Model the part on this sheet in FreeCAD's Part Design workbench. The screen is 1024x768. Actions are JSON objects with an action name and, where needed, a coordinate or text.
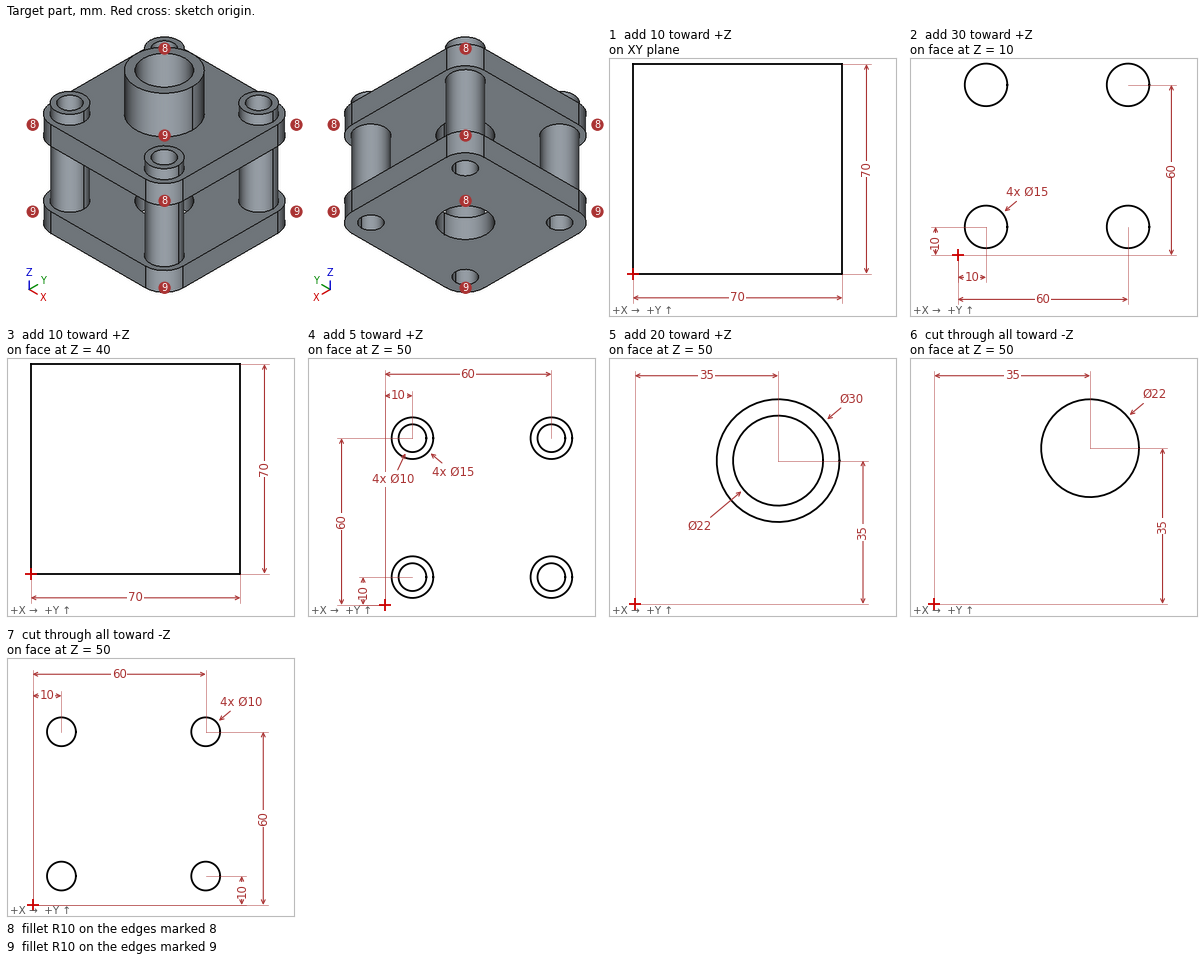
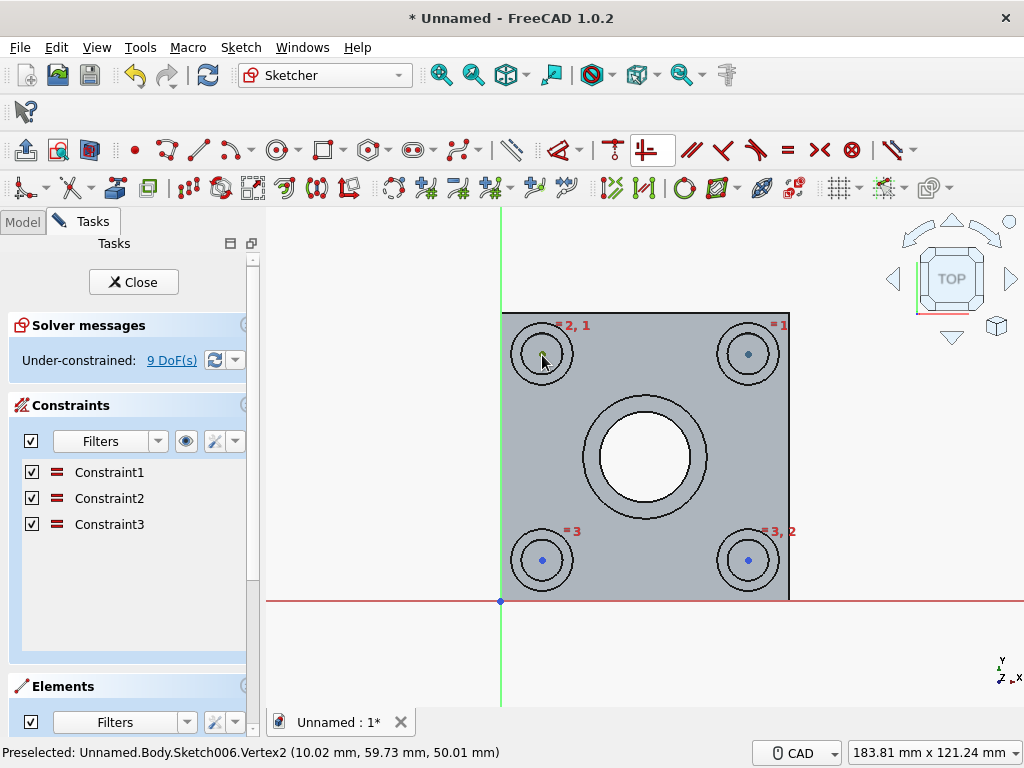
{"action": "key", "text": "h"}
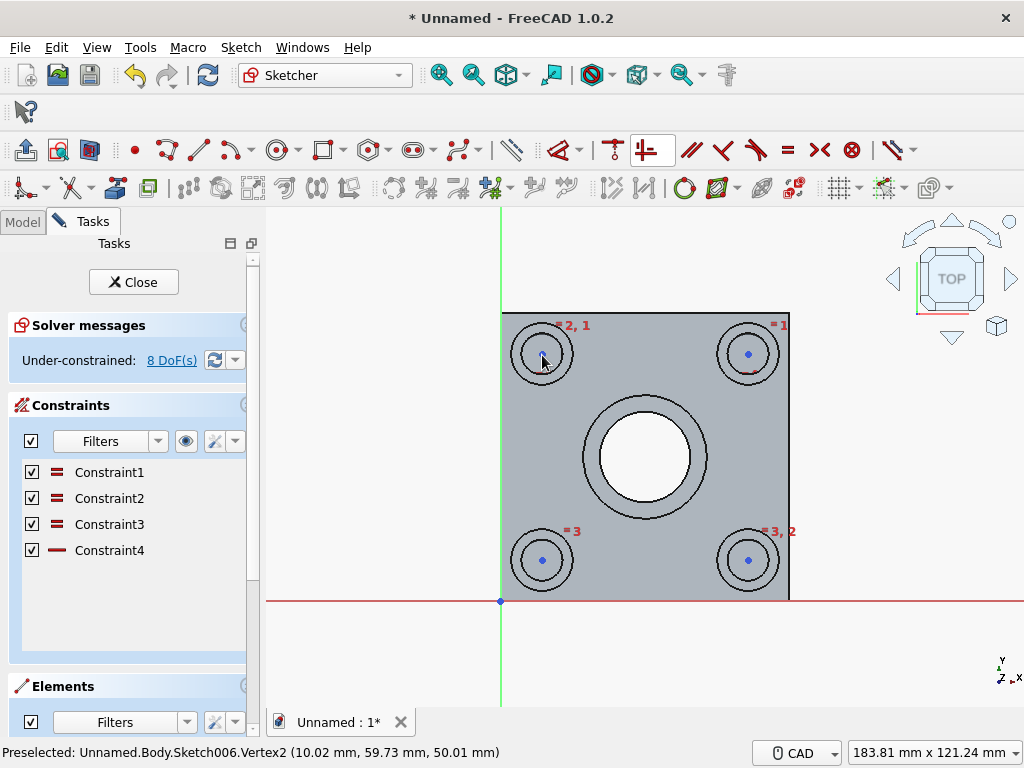
{"action": "left_click", "coordinate": [748, 355]}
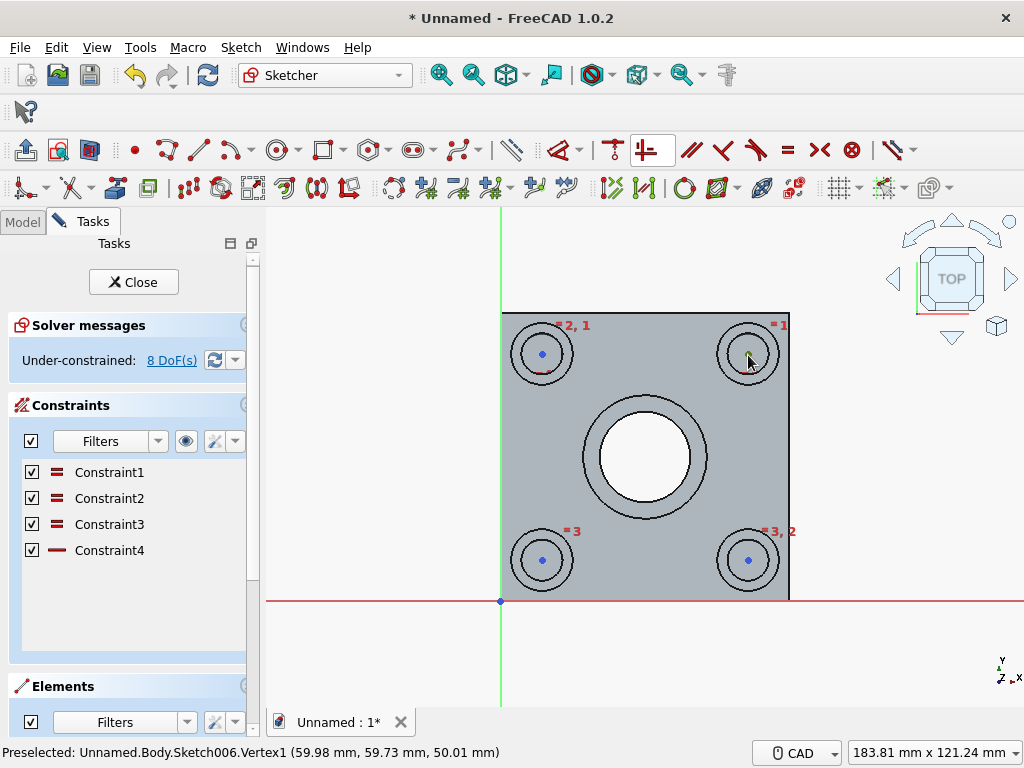
{"action": "left_click", "coordinate": [748, 561]}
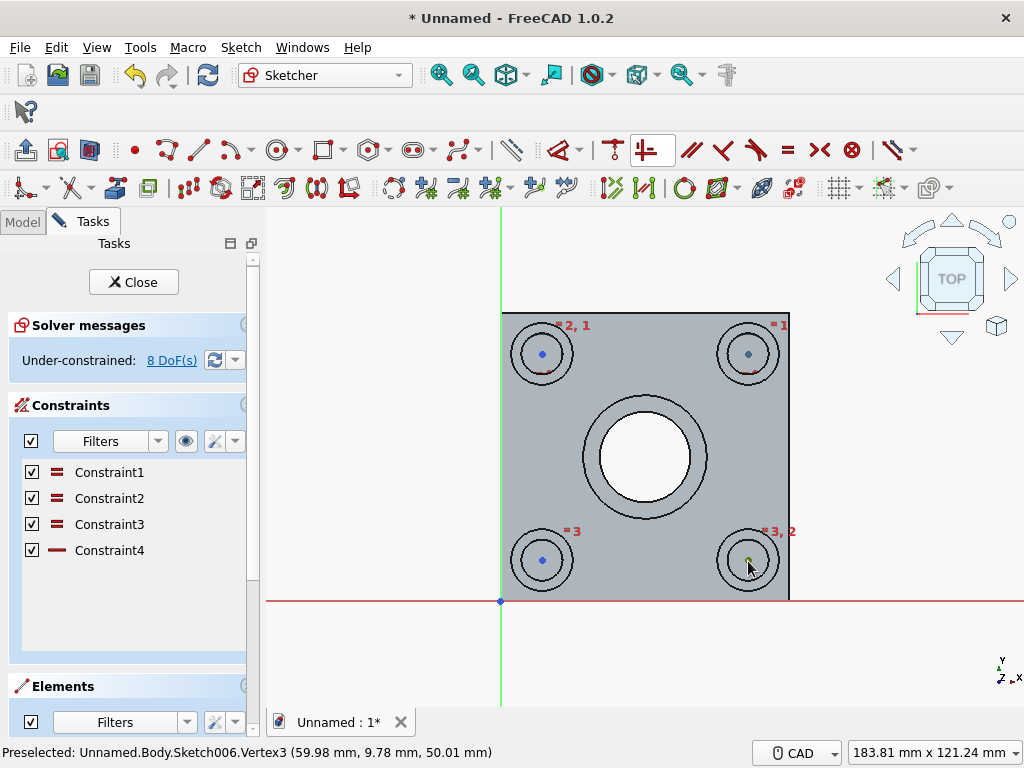
{"action": "key", "text": "v"}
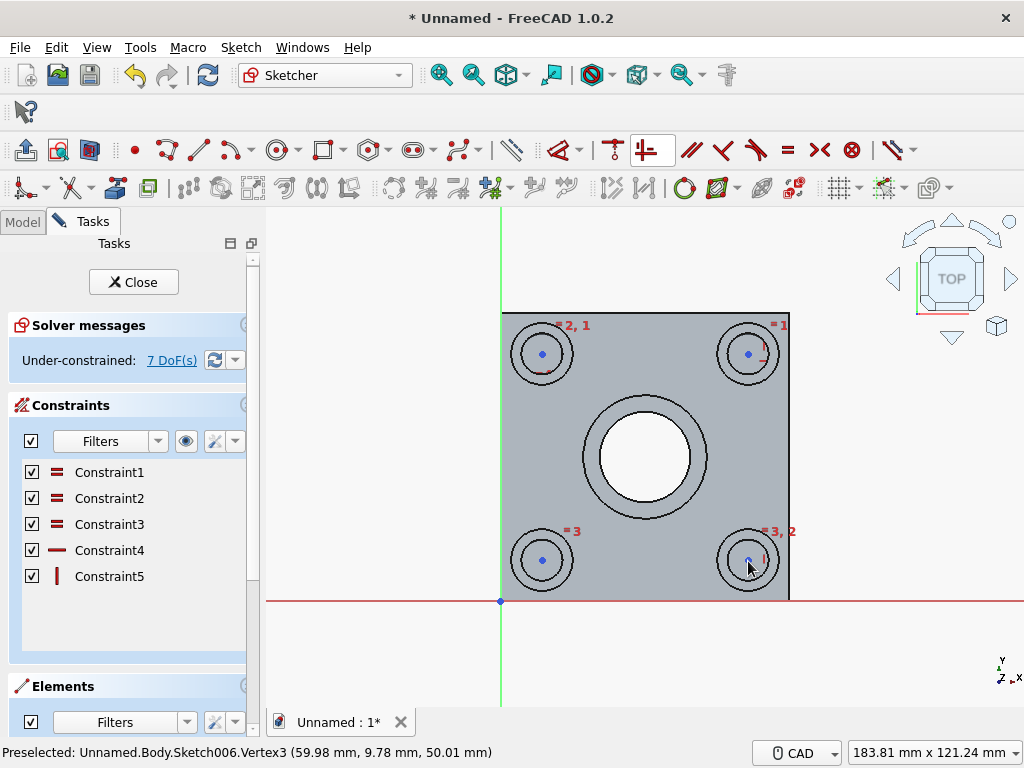
{"action": "left_click", "coordinate": [542, 355]}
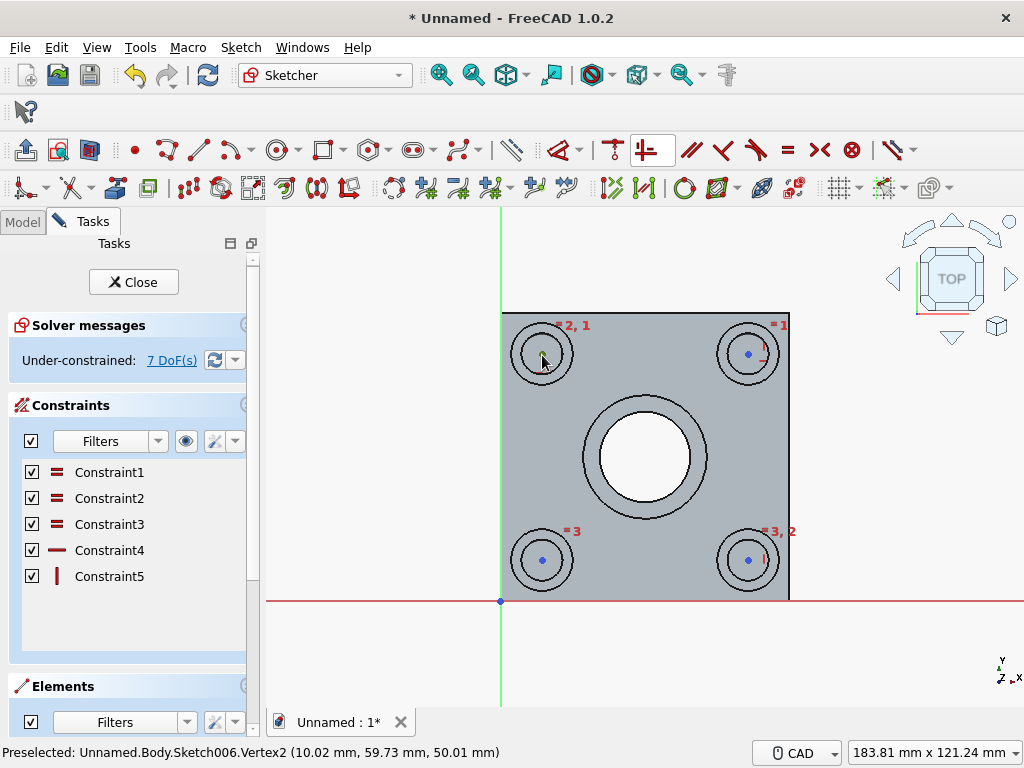
{"action": "left_click", "coordinate": [542, 561]}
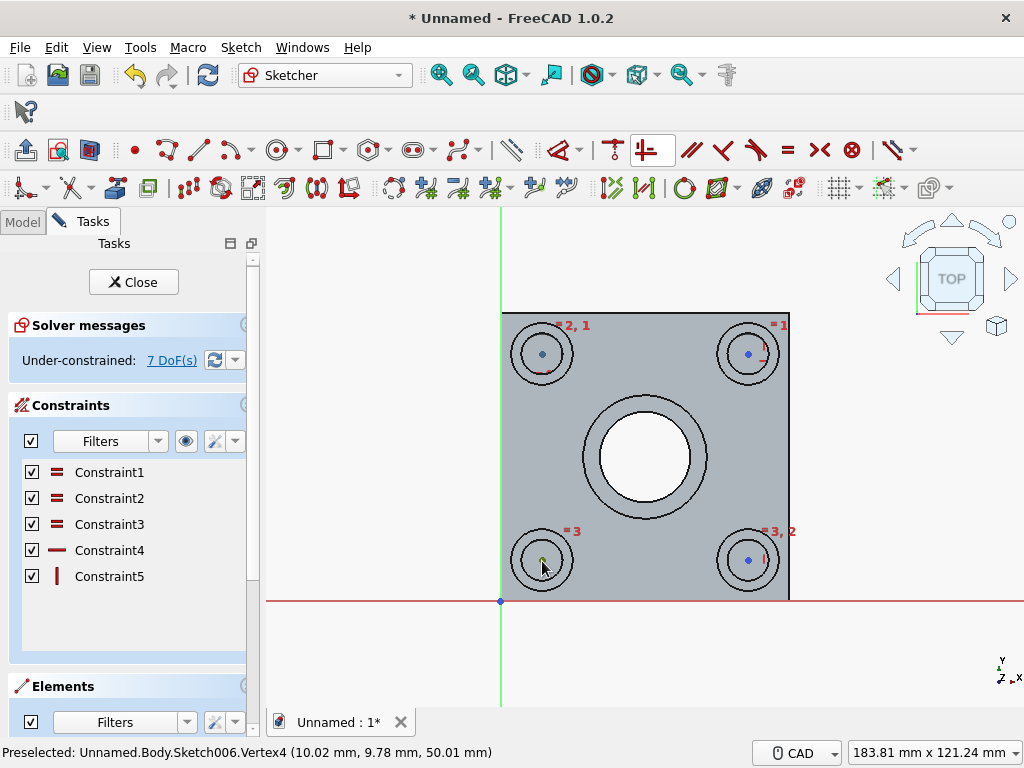
{"action": "key", "text": "v"}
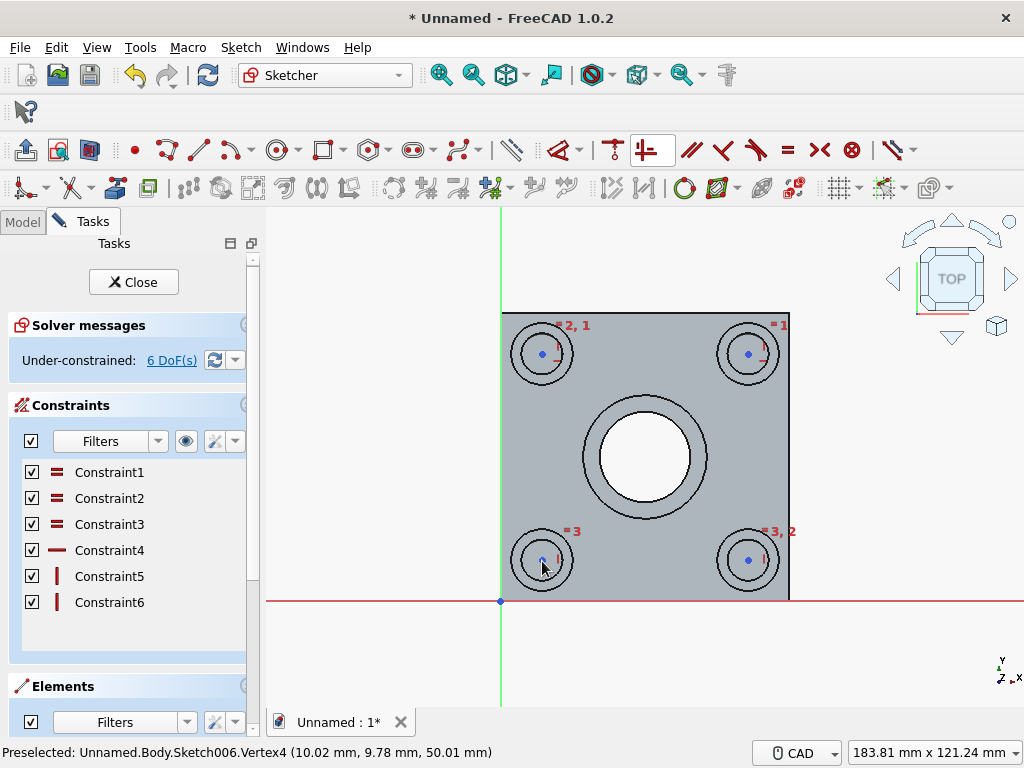
{"action": "left_click", "coordinate": [748, 561]}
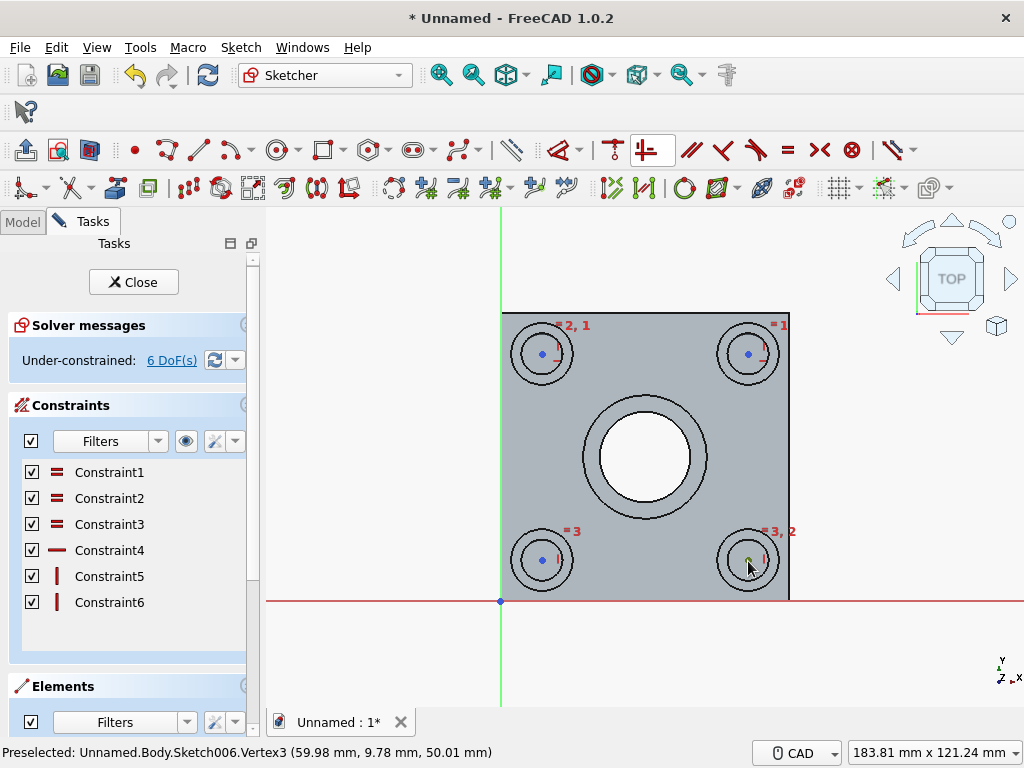
{"action": "left_click", "coordinate": [542, 561]}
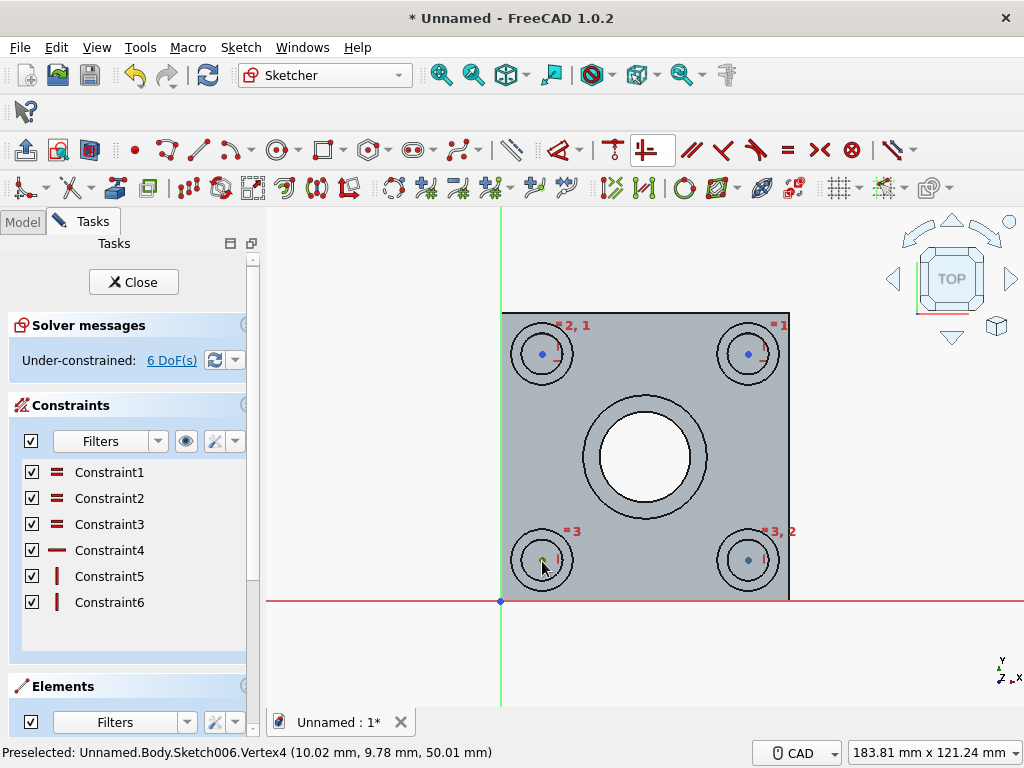
{"action": "key", "text": "h"}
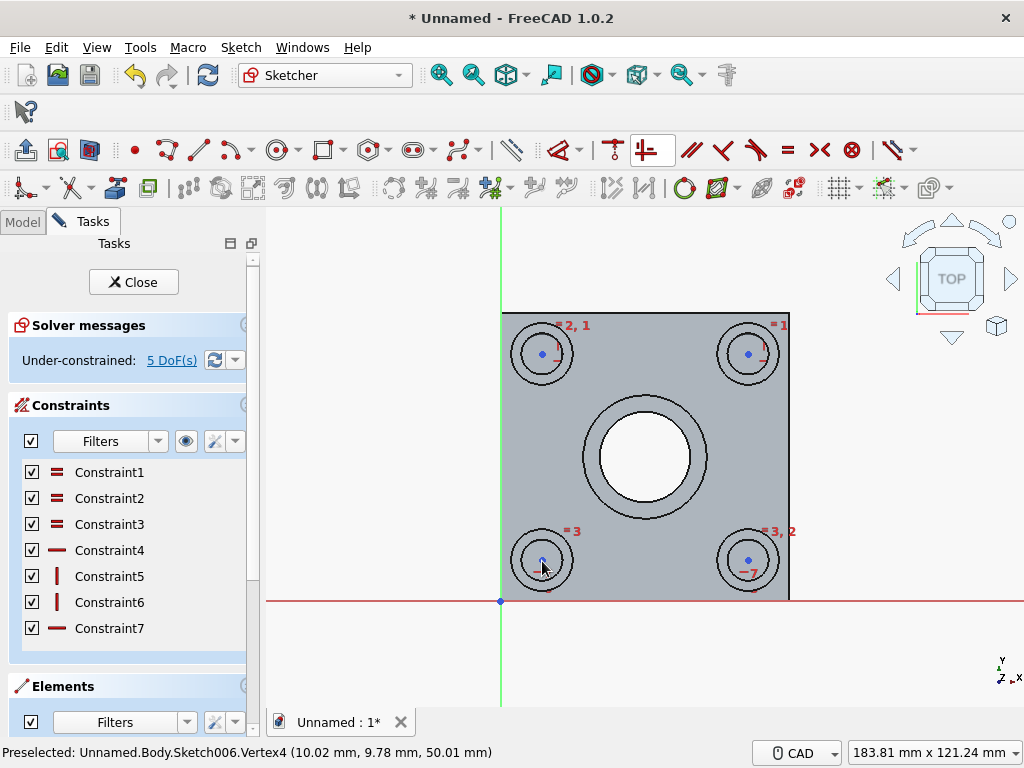
{"action": "left_click", "coordinate": [558, 150]}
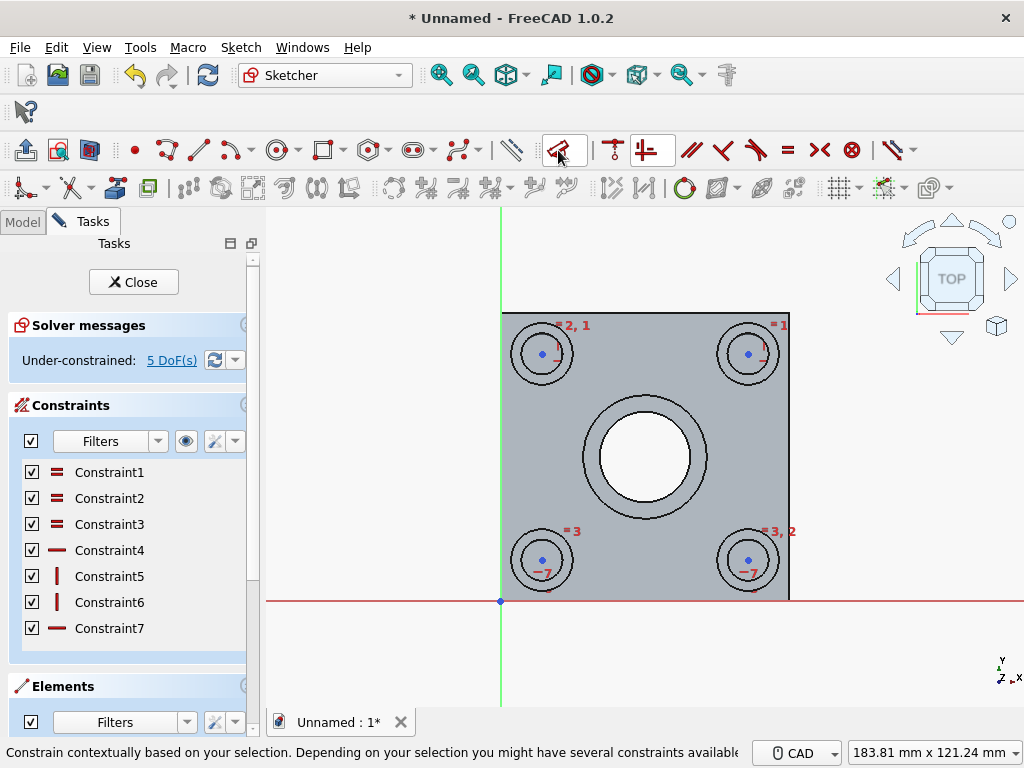
{"action": "left_click", "coordinate": [763, 340]}
{"action": "left_click", "coordinate": [786, 317]}